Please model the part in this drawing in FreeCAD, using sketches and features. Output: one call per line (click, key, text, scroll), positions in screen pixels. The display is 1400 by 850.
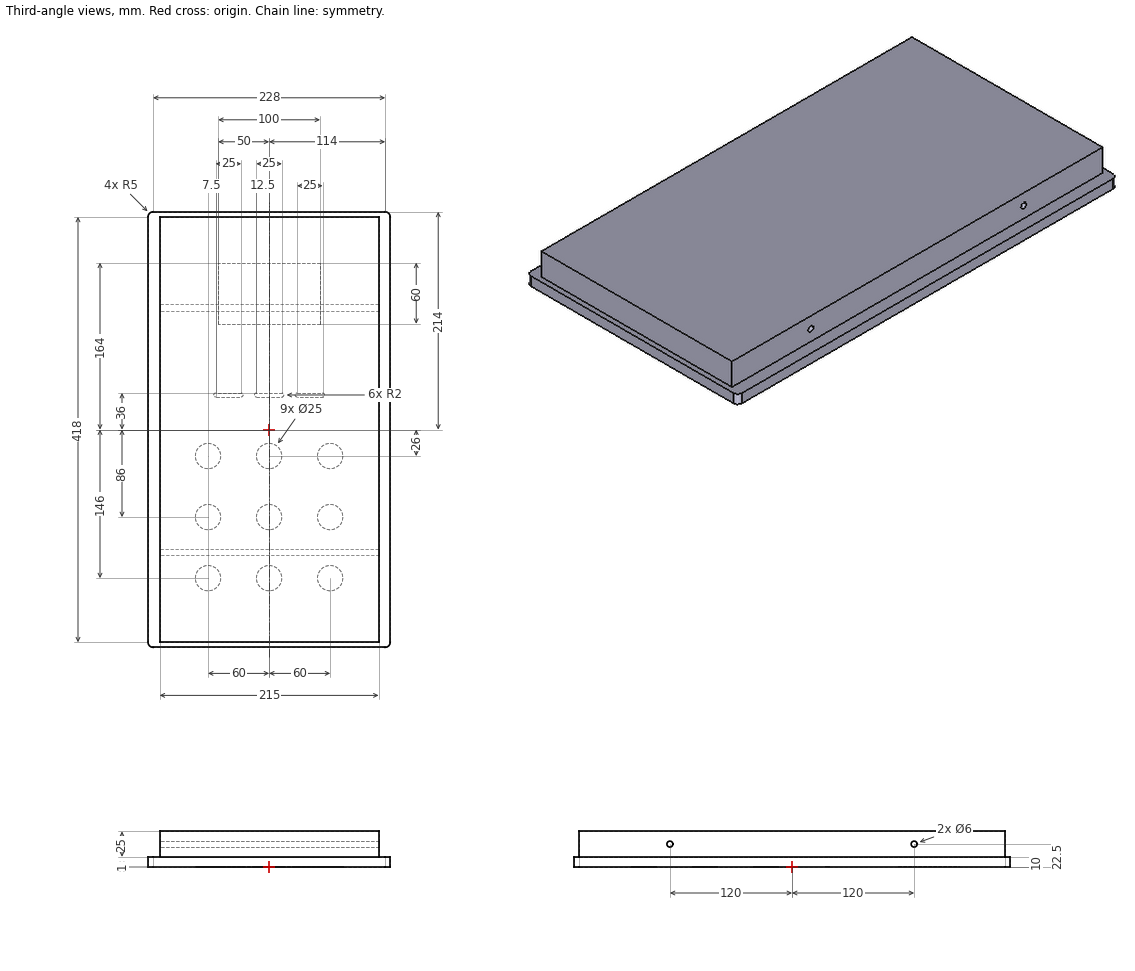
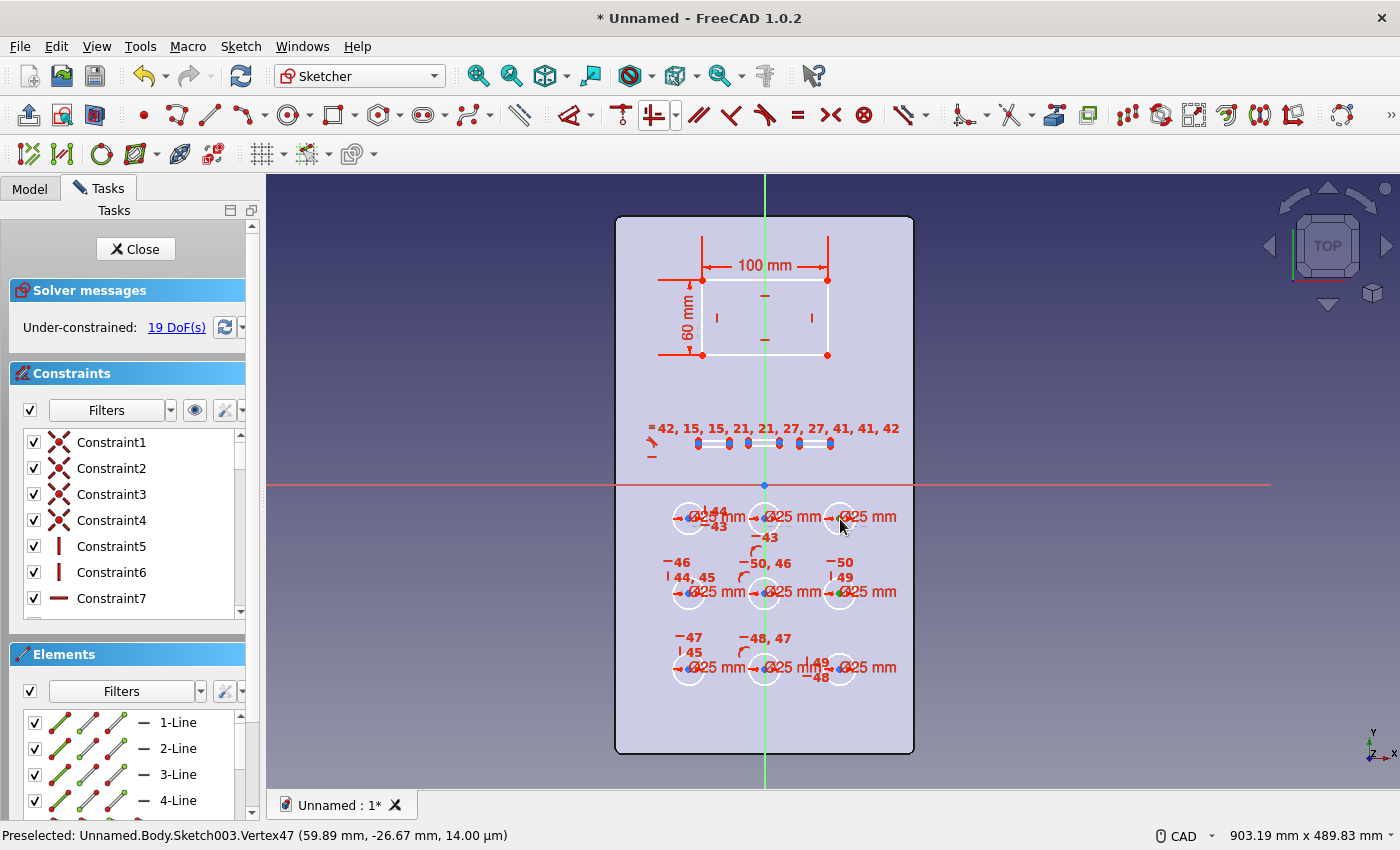
key(v)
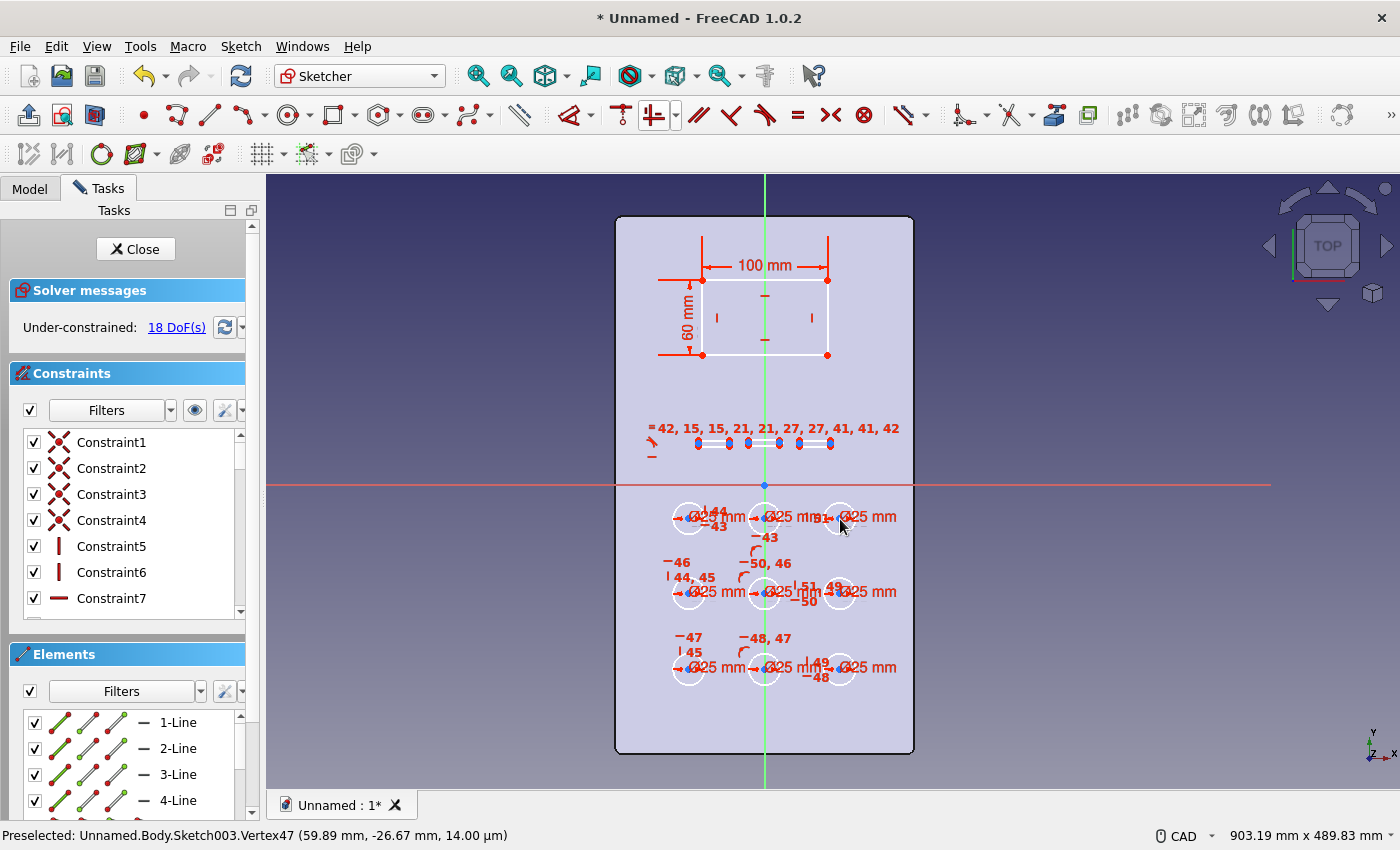
click(765, 519)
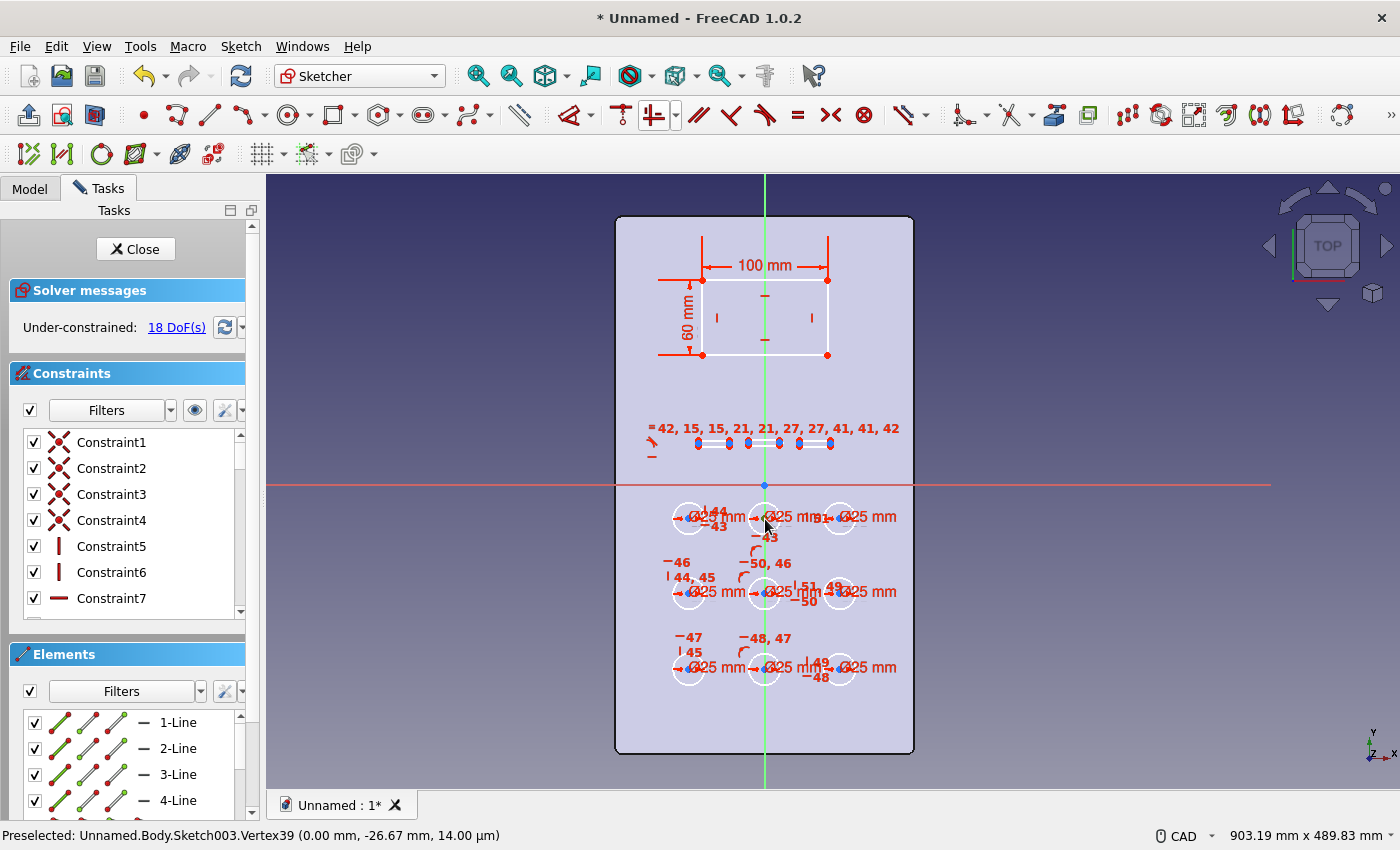
click(840, 519)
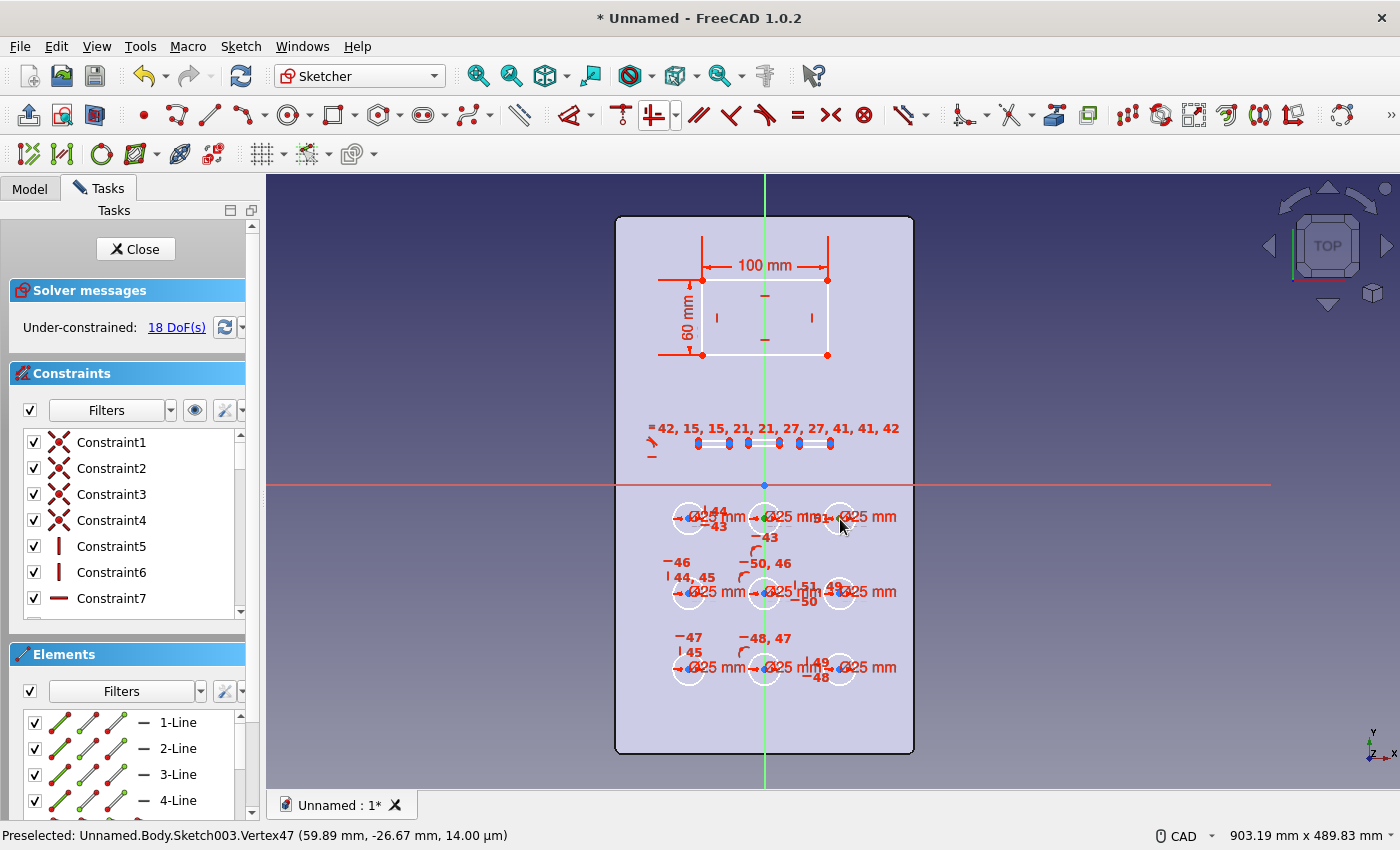
click(676, 116)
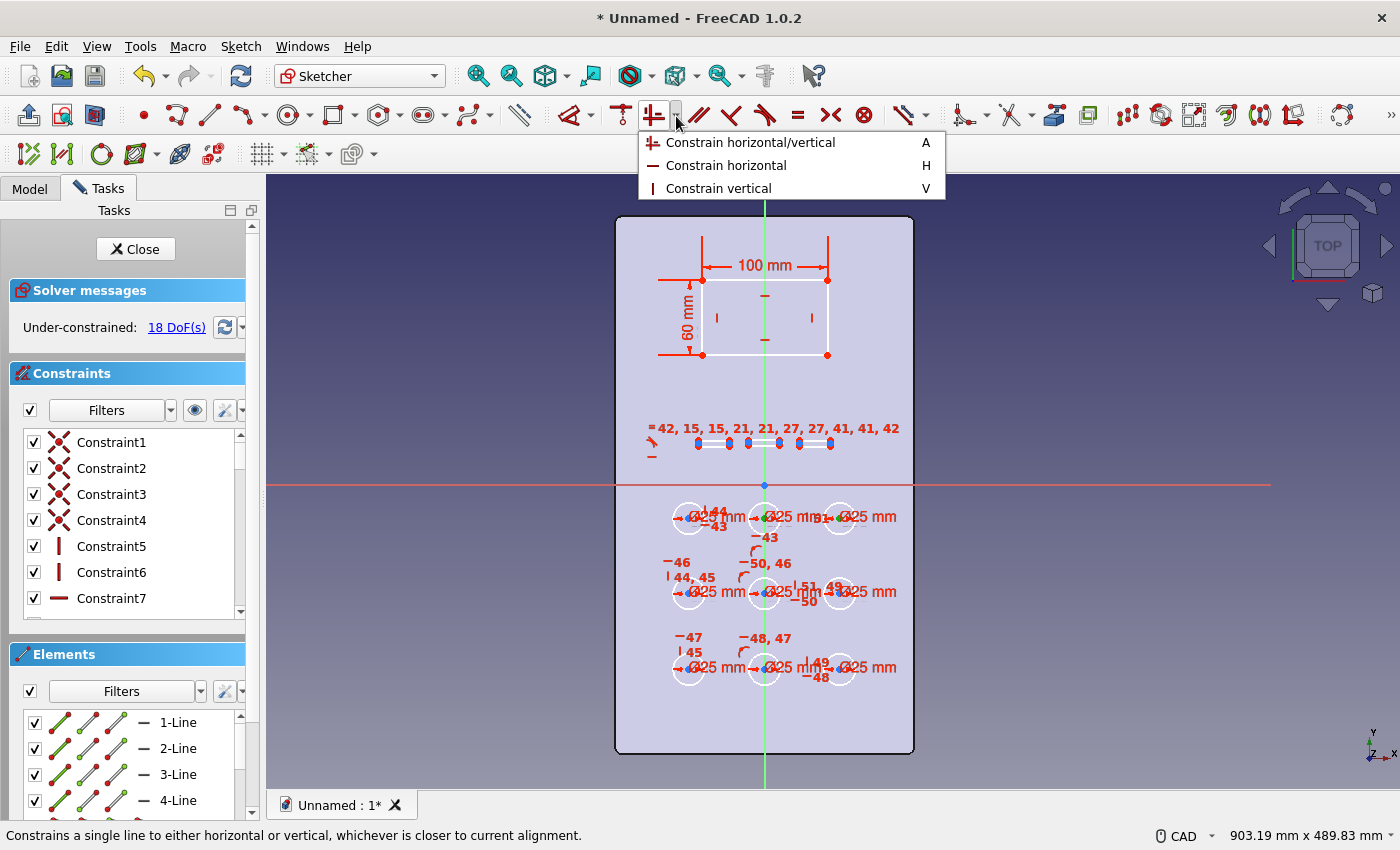
click(792, 166)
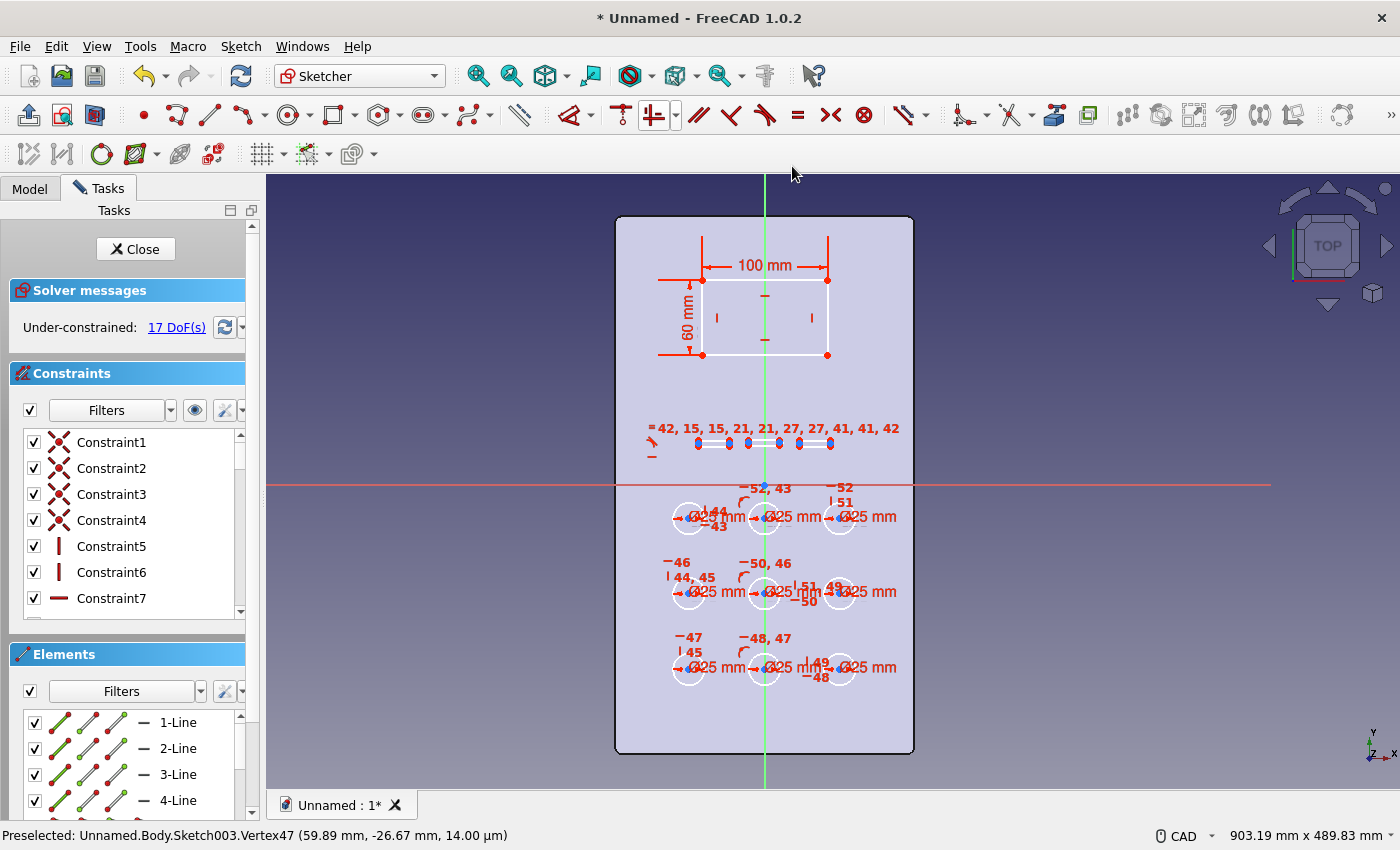
scroll(730, 444, up, 8)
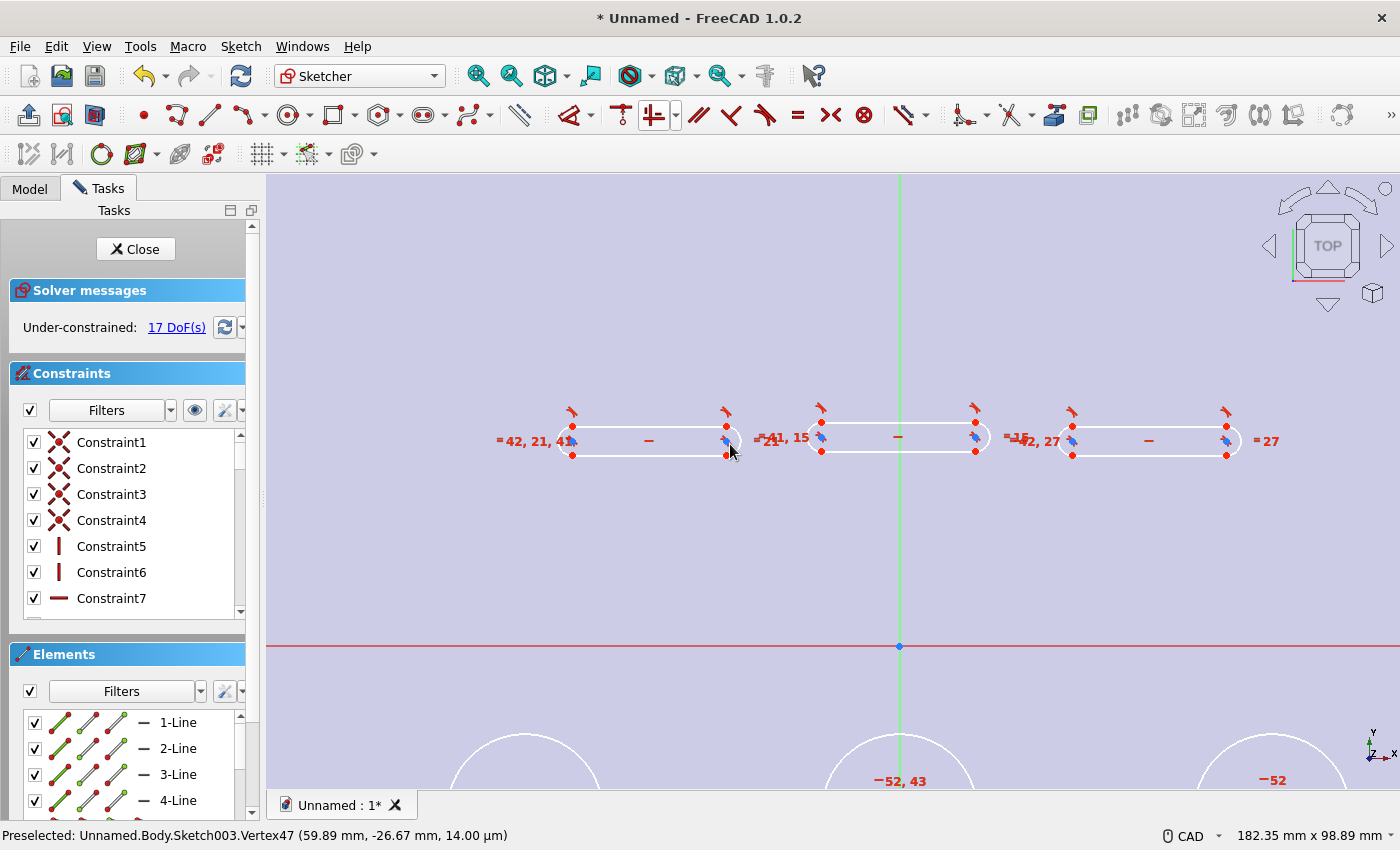
click(726, 441)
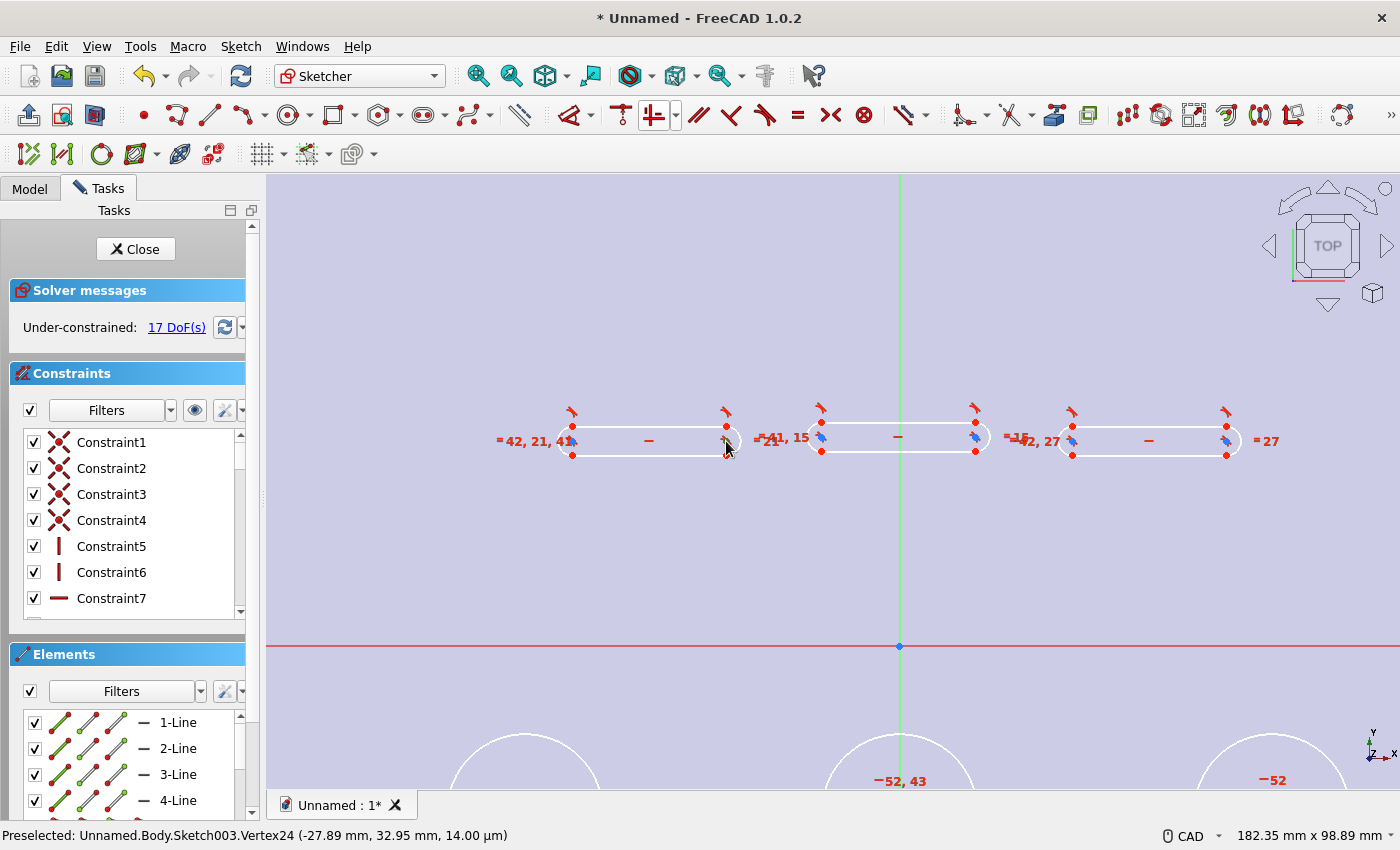
click(1073, 441)